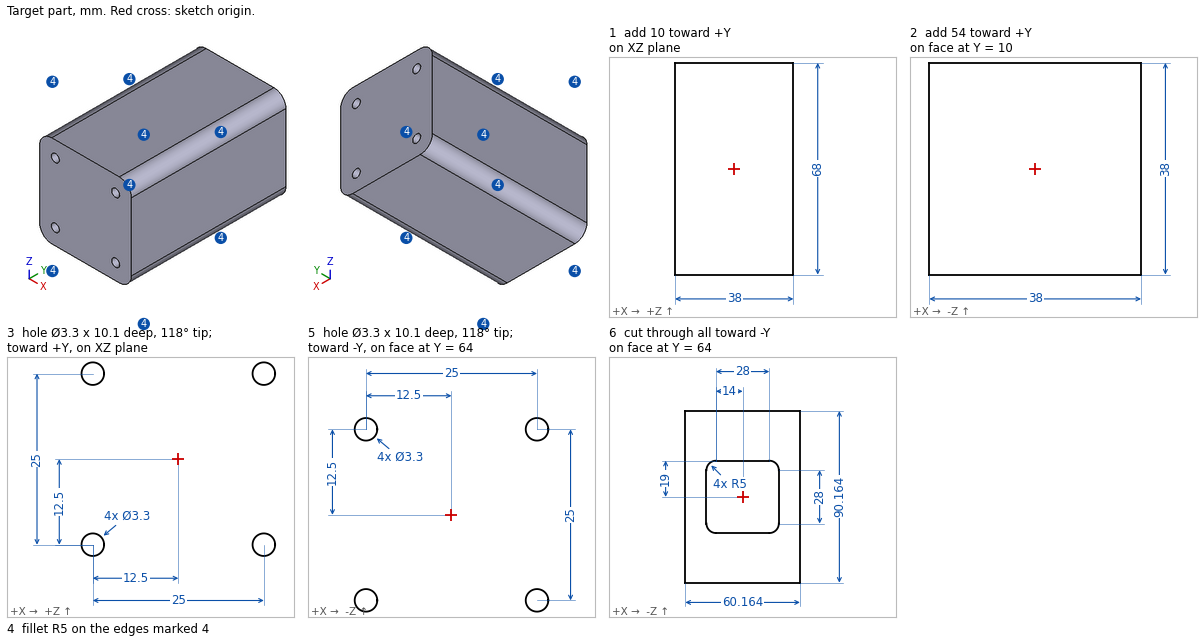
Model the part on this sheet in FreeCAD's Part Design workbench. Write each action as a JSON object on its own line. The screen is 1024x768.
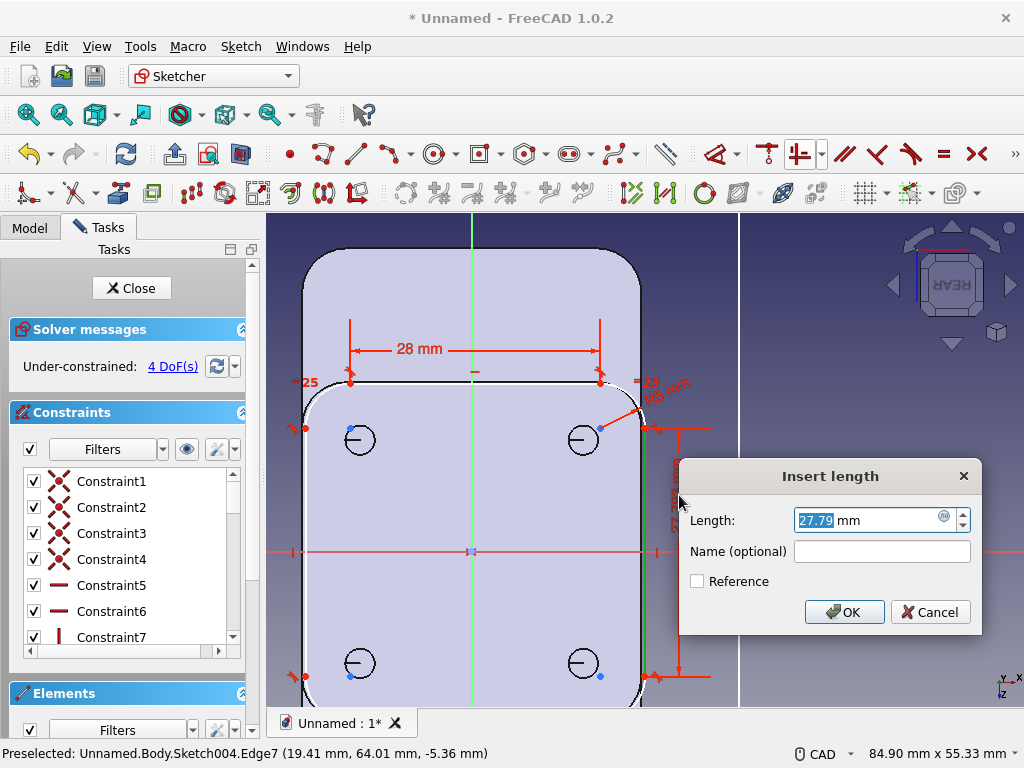
{"action": "type", "text": "28"}
{"action": "key", "text": "Return"}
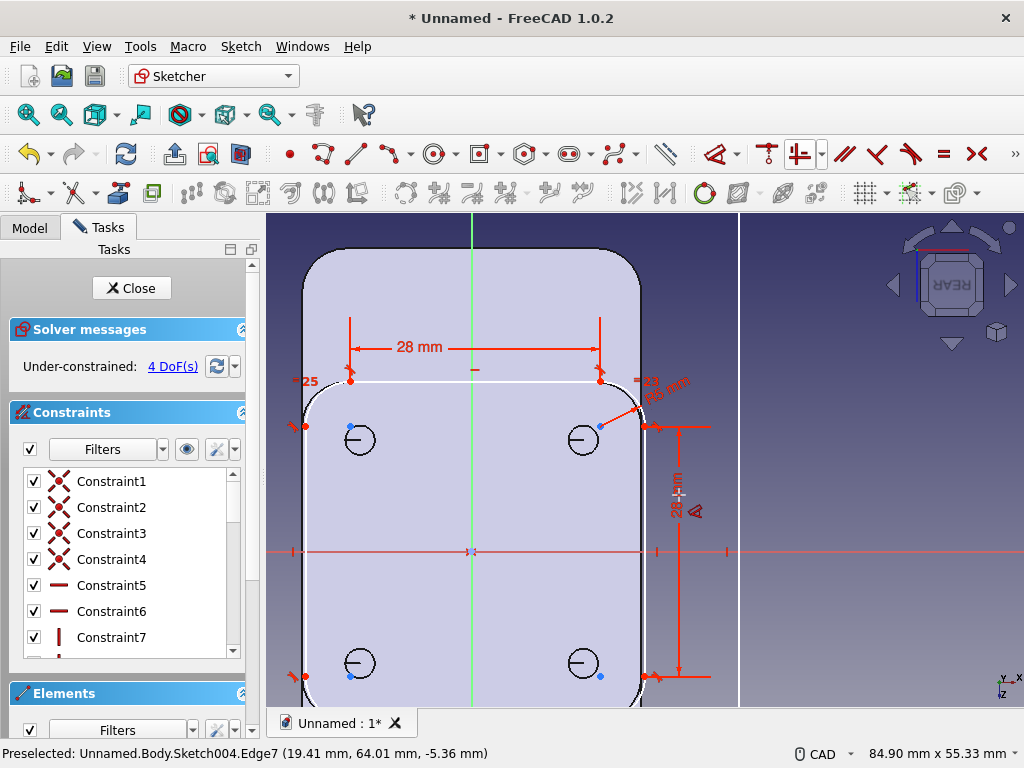
{"action": "left_click", "coordinate": [350, 382]}
{"action": "left_click", "coordinate": [411, 586]}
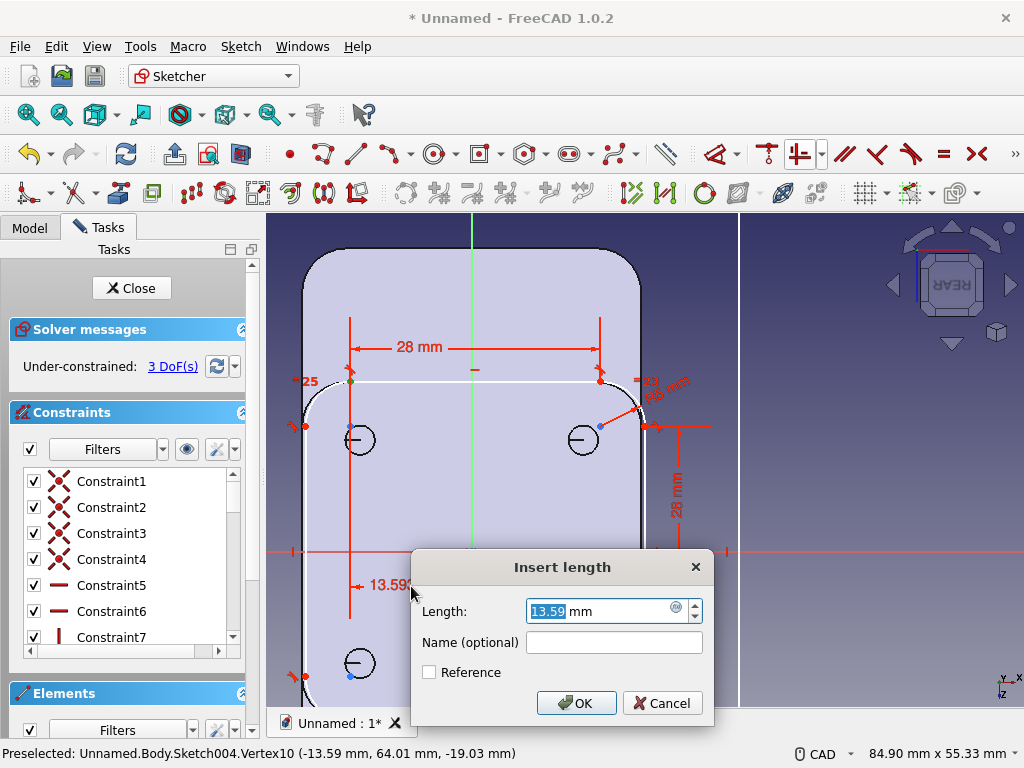
{"action": "type", "text": "14"}
{"action": "key", "text": "Return"}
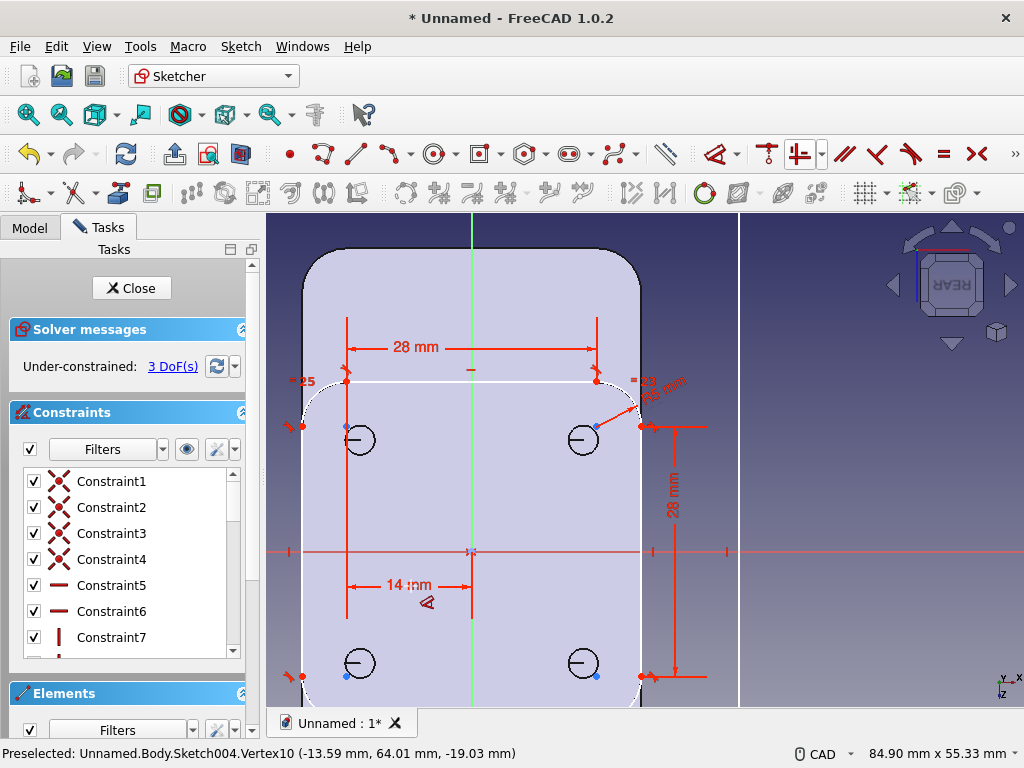
{"action": "left_click", "coordinate": [347, 382]}
{"action": "left_click", "coordinate": [506, 467]}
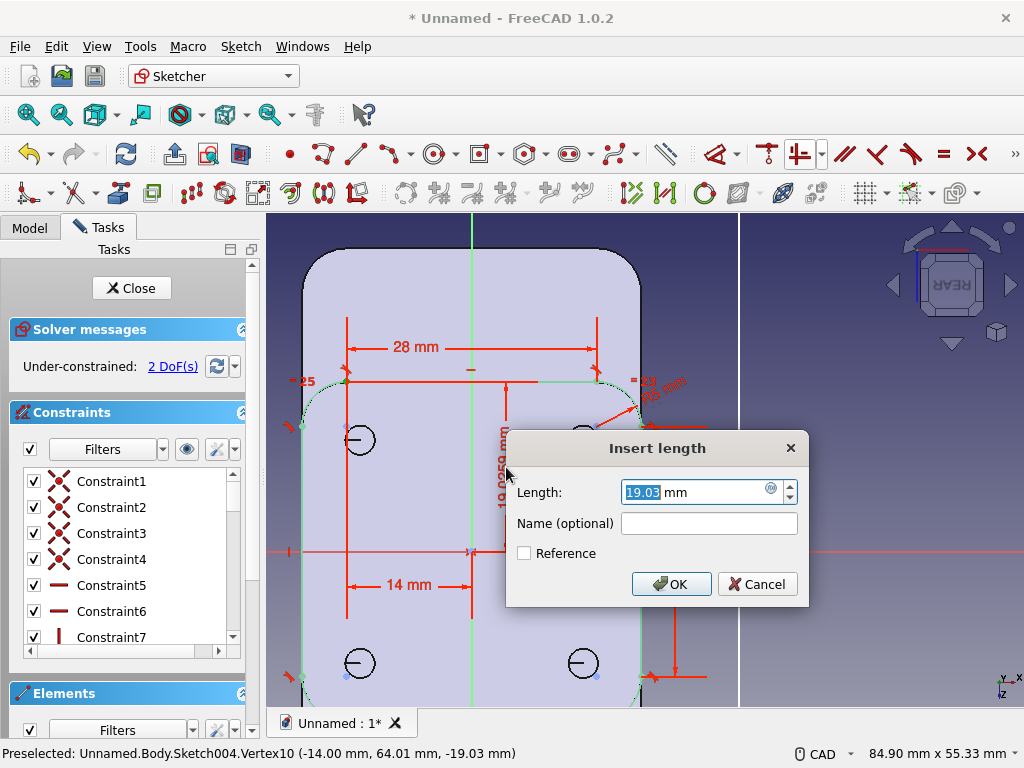
{"action": "type", "text": "19"}
{"action": "key", "text": "Return"}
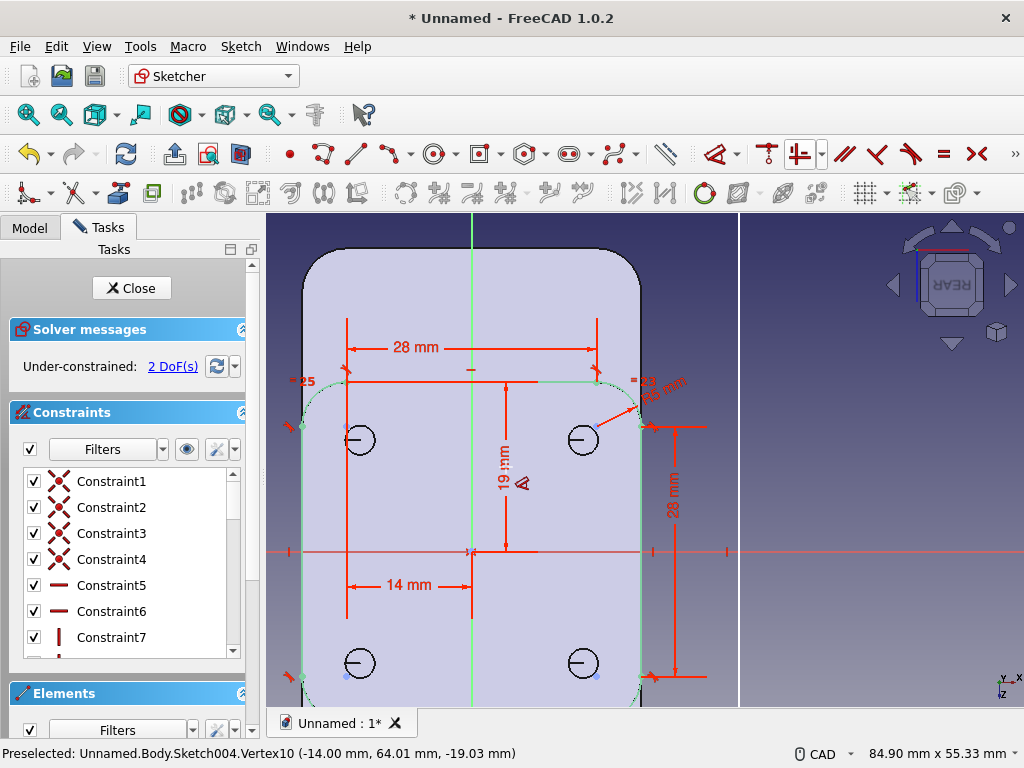
{"action": "scroll", "coordinate": [637, 407], "scroll_direction": "down", "scroll_amount": 5}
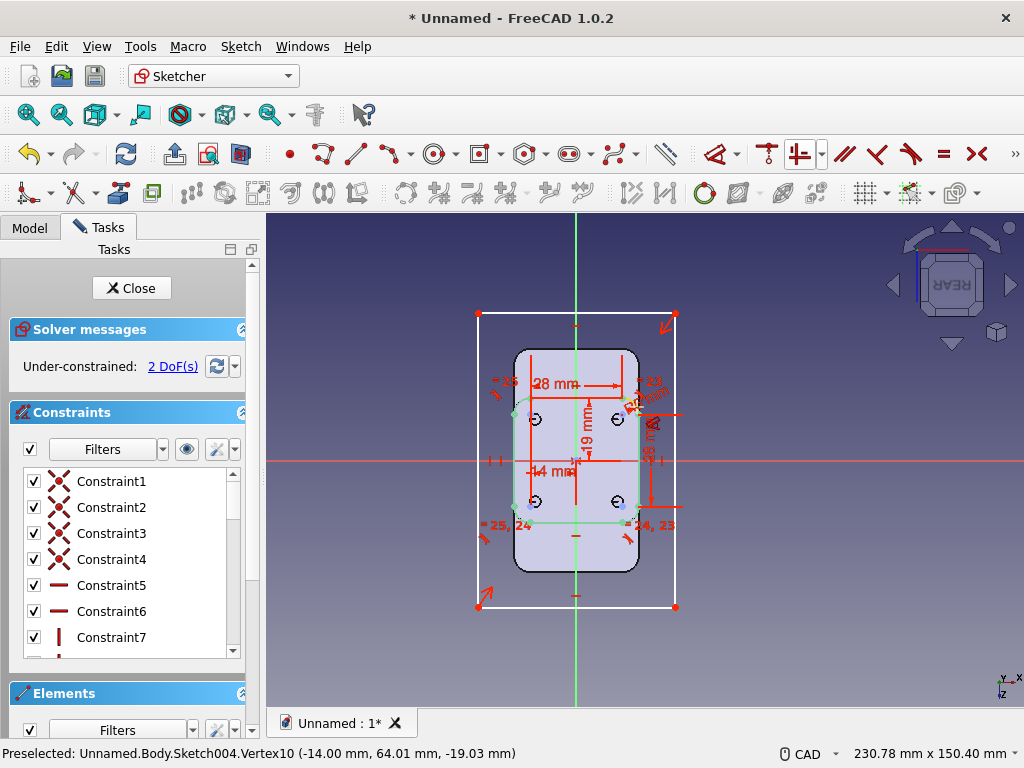
{"action": "left_click", "coordinate": [537, 608]}
{"action": "left_click", "coordinate": [531, 642]}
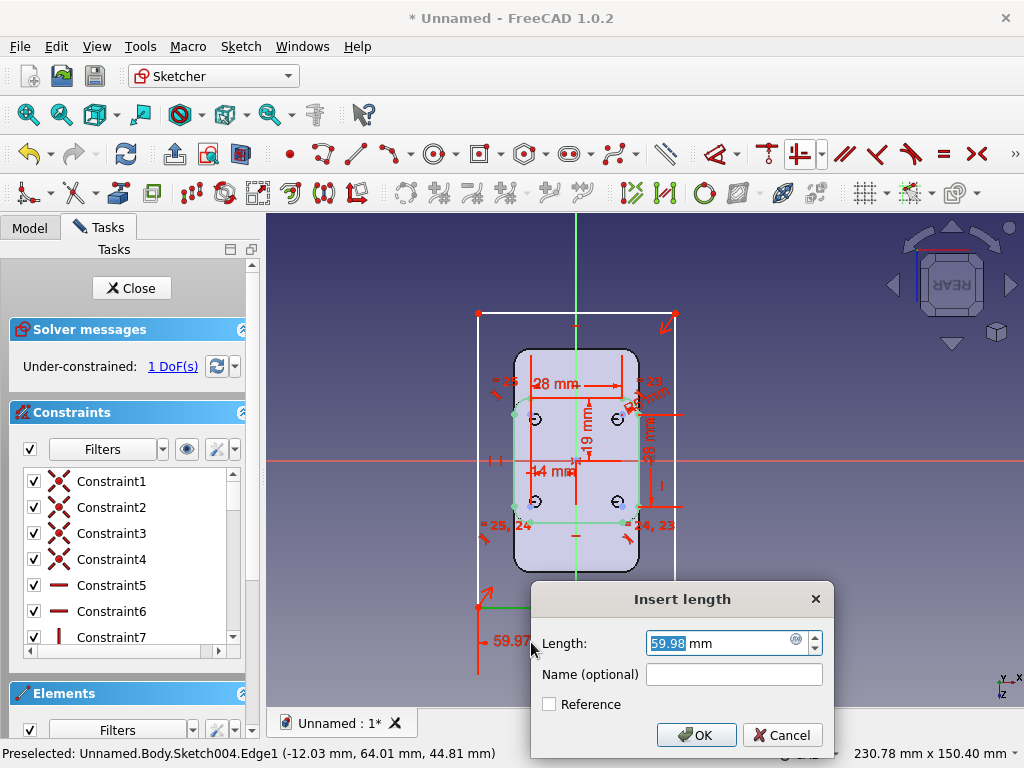
{"action": "type", "text": "60.164"}
{"action": "key", "text": "Return"}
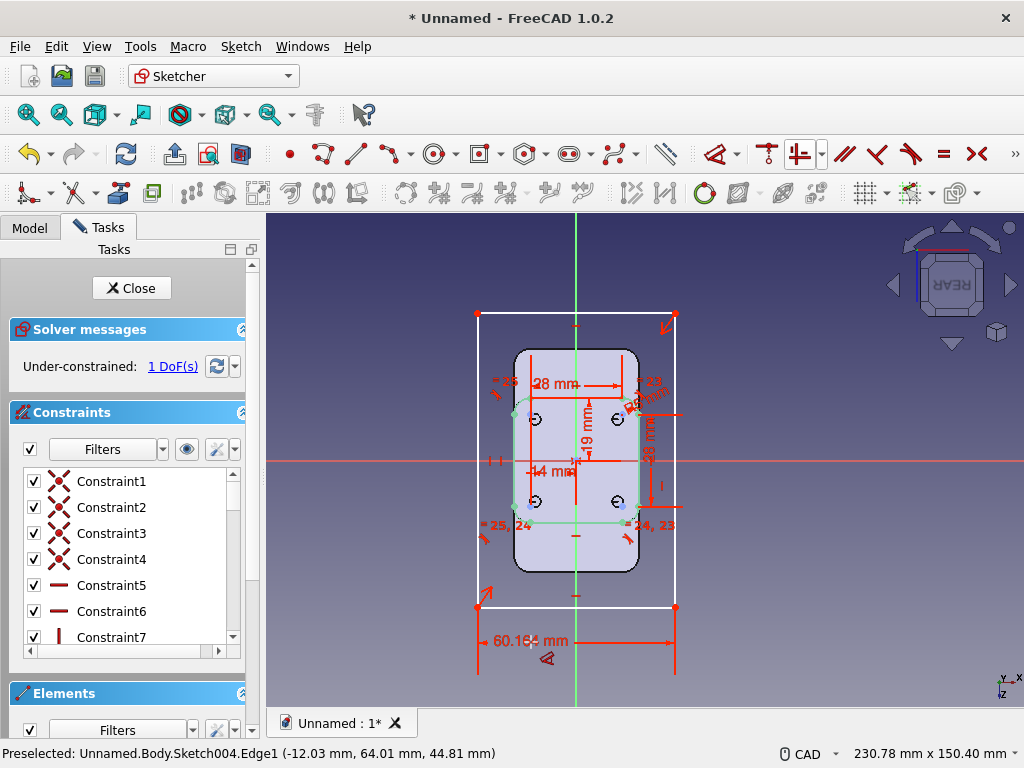
{"action": "left_click", "coordinate": [675, 519]}
{"action": "left_click", "coordinate": [709, 528]}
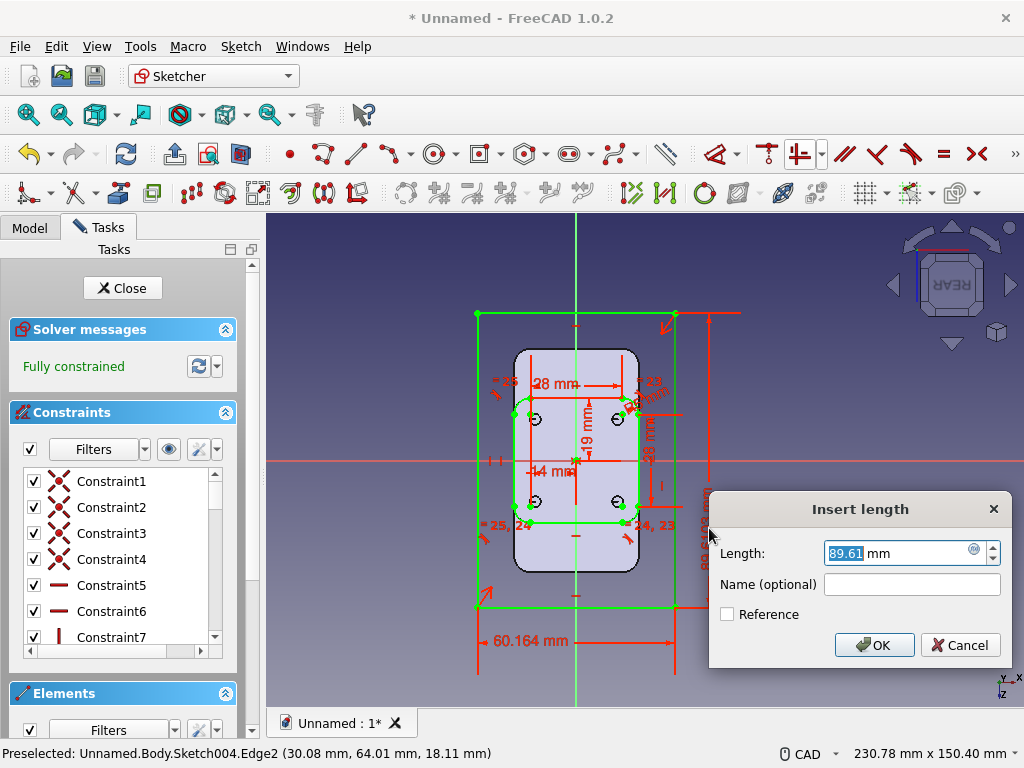
{"action": "type", "text": "90.164"}
{"action": "key", "text": "Return"}
{"action": "key", "text": "Escape"}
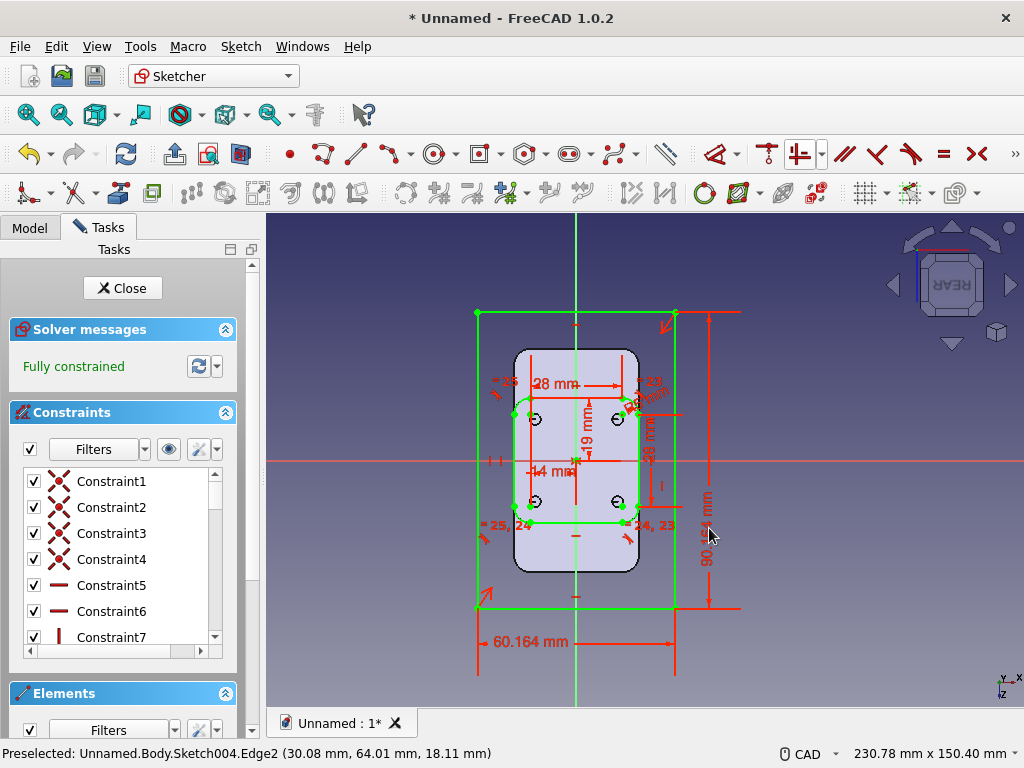
{"action": "left_click", "coordinate": [123, 288]}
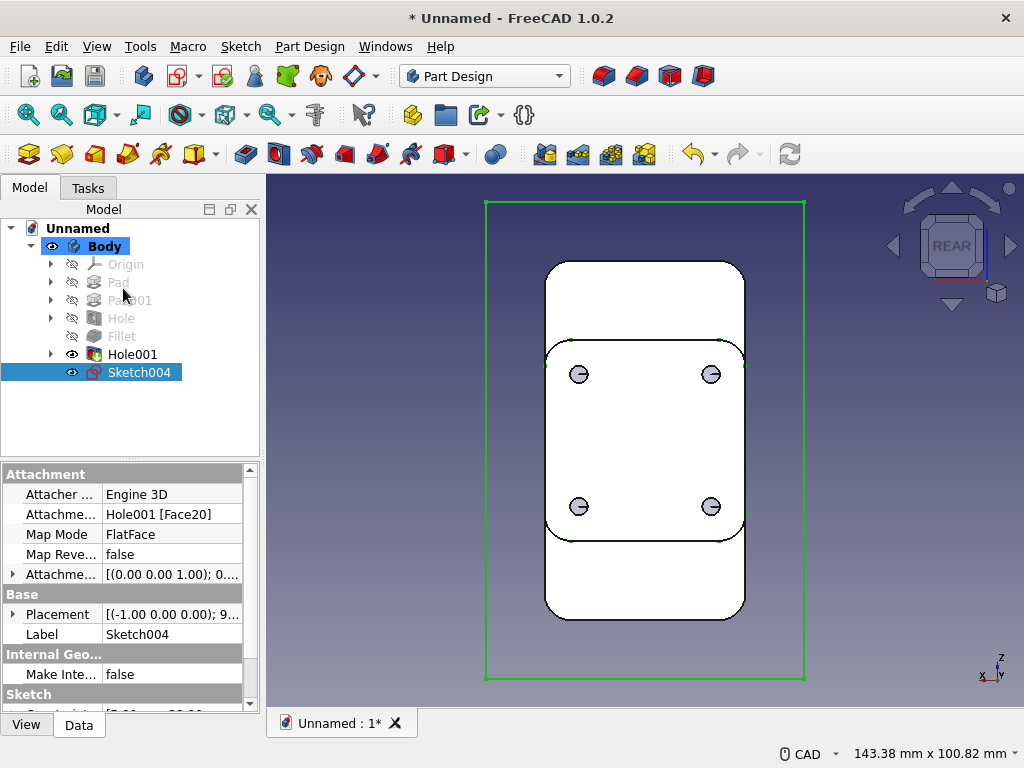
{"action": "left_click", "coordinate": [246, 154]}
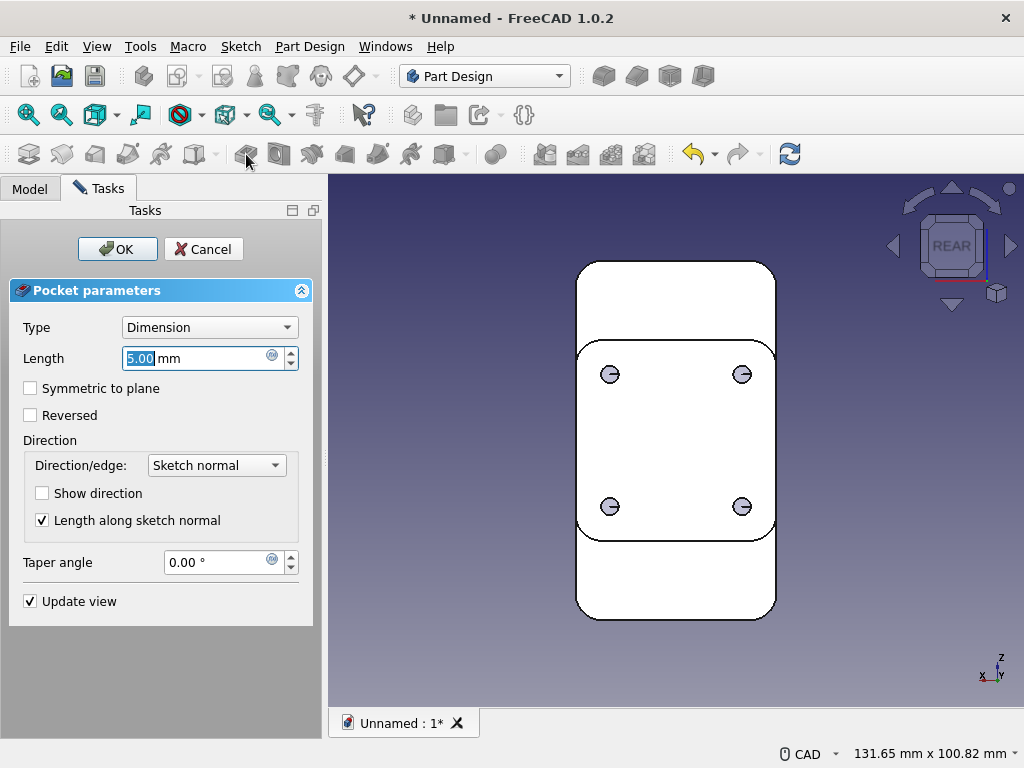
{"action": "left_click", "coordinate": [210, 328]}